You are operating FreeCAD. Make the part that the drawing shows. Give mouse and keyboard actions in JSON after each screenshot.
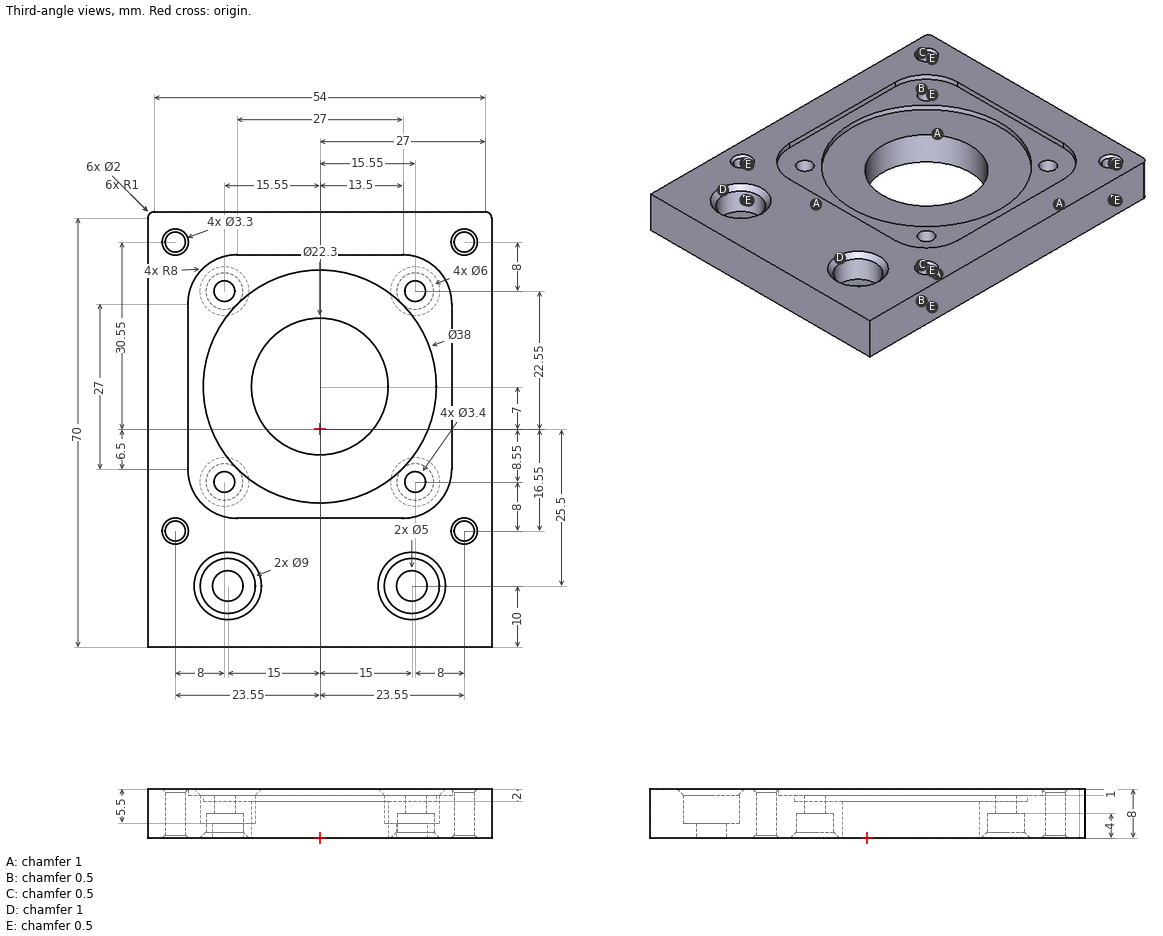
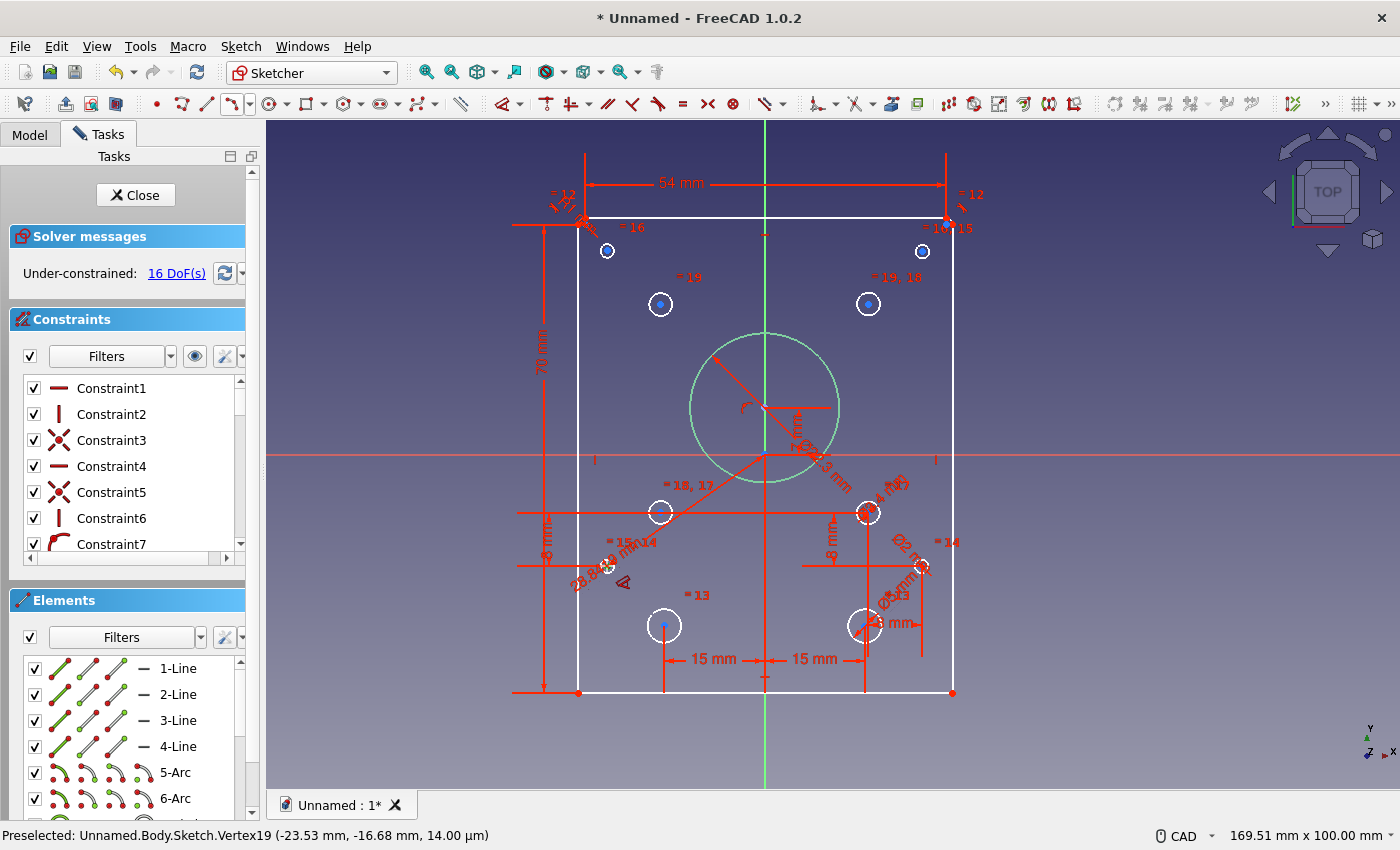
{"action": "left_click", "coordinate": [661, 512]}
{"action": "left_click", "coordinate": [634, 600]}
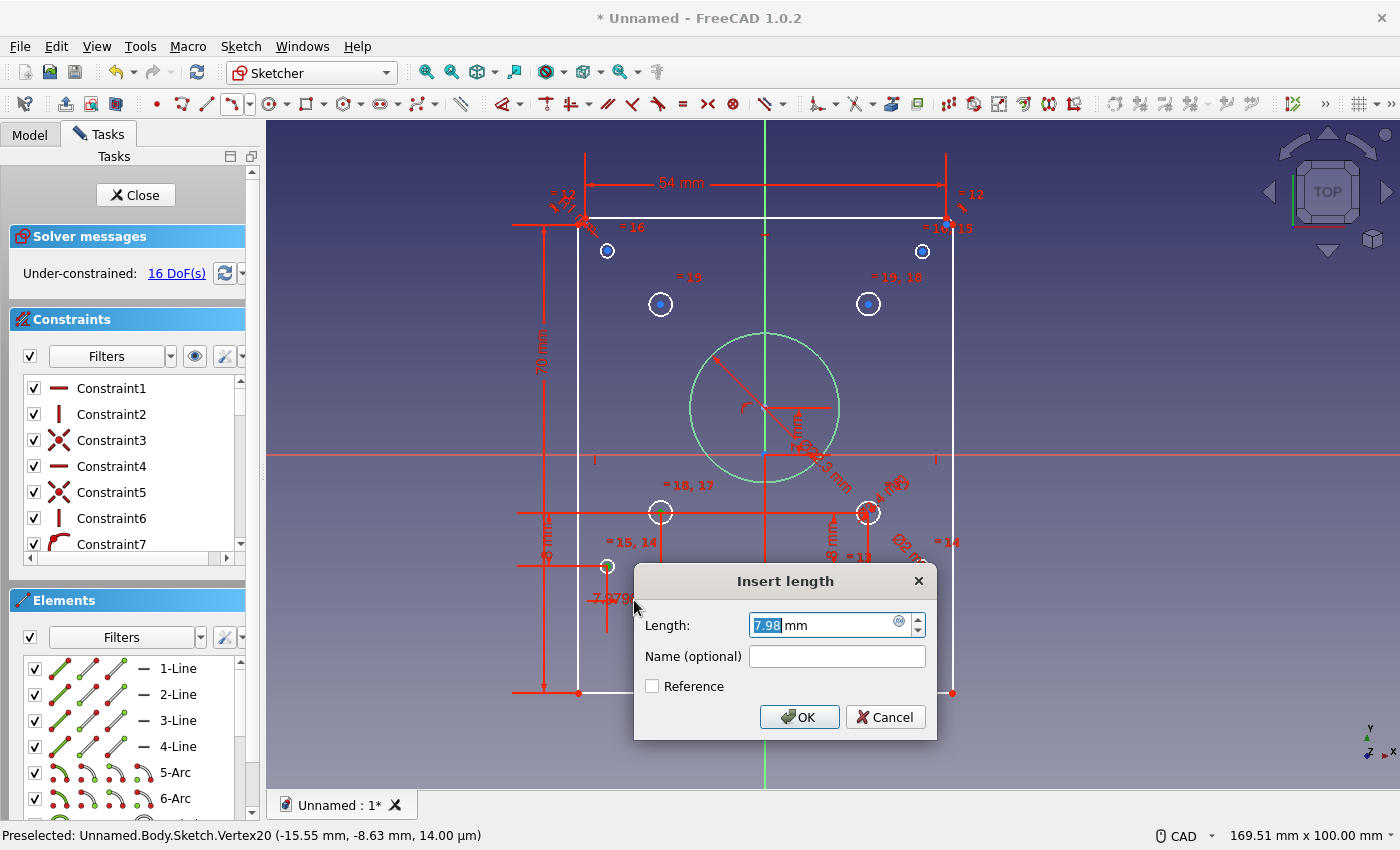
{"action": "type", "text": "8"}
{"action": "key", "text": "Return"}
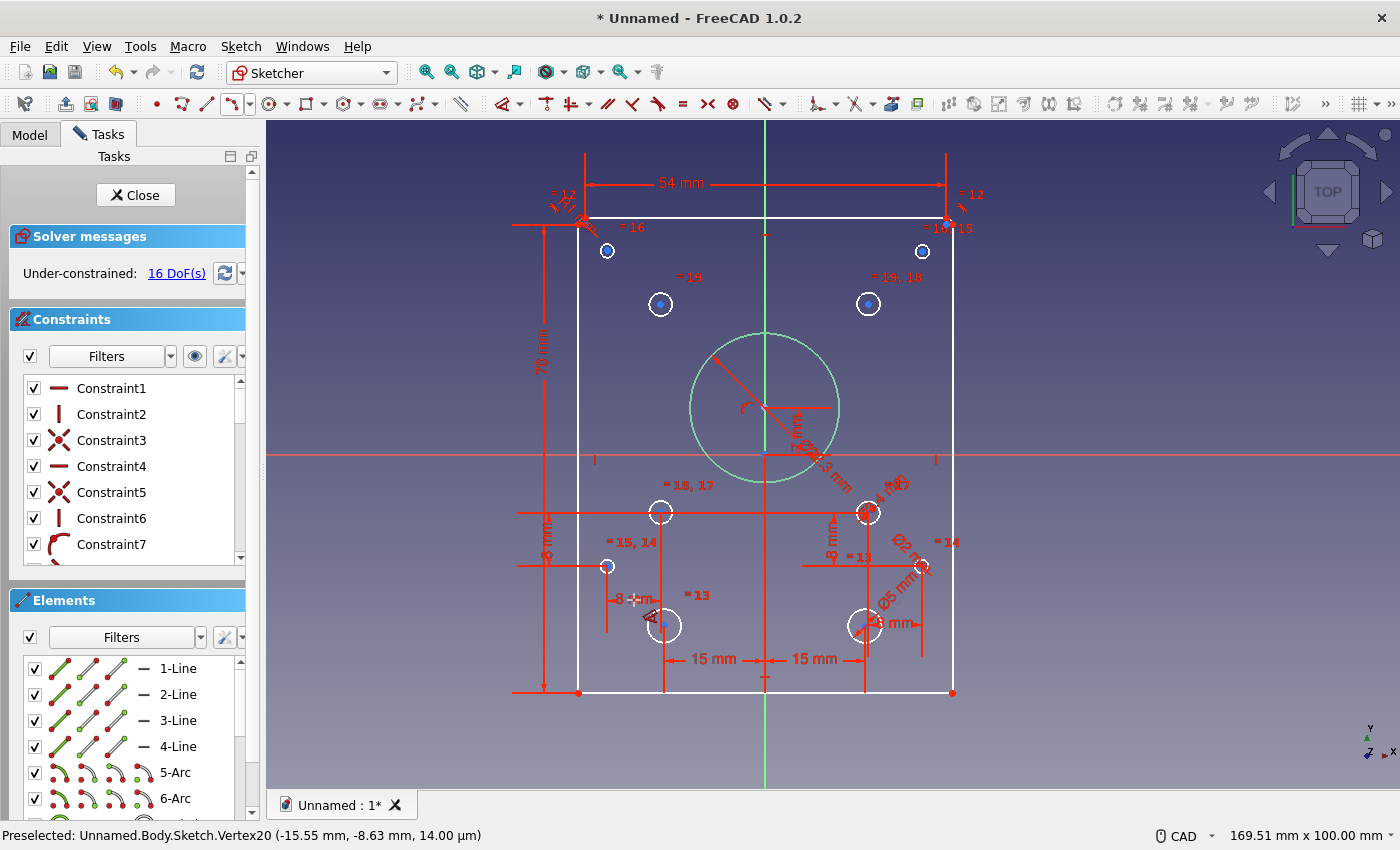
{"action": "left_click", "coordinate": [607, 566]}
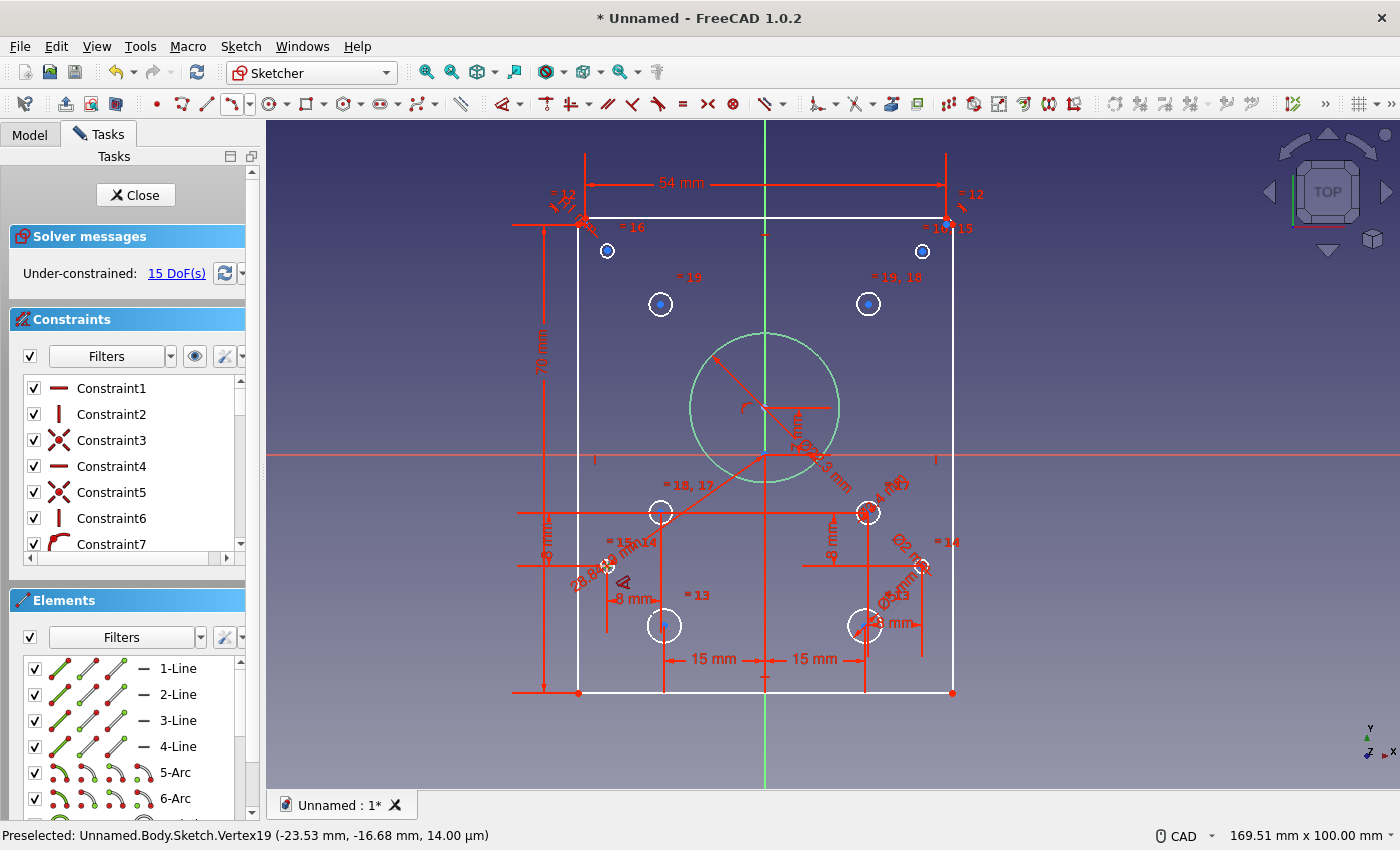
{"action": "left_click", "coordinate": [661, 512]}
{"action": "left_click", "coordinate": [695, 539]}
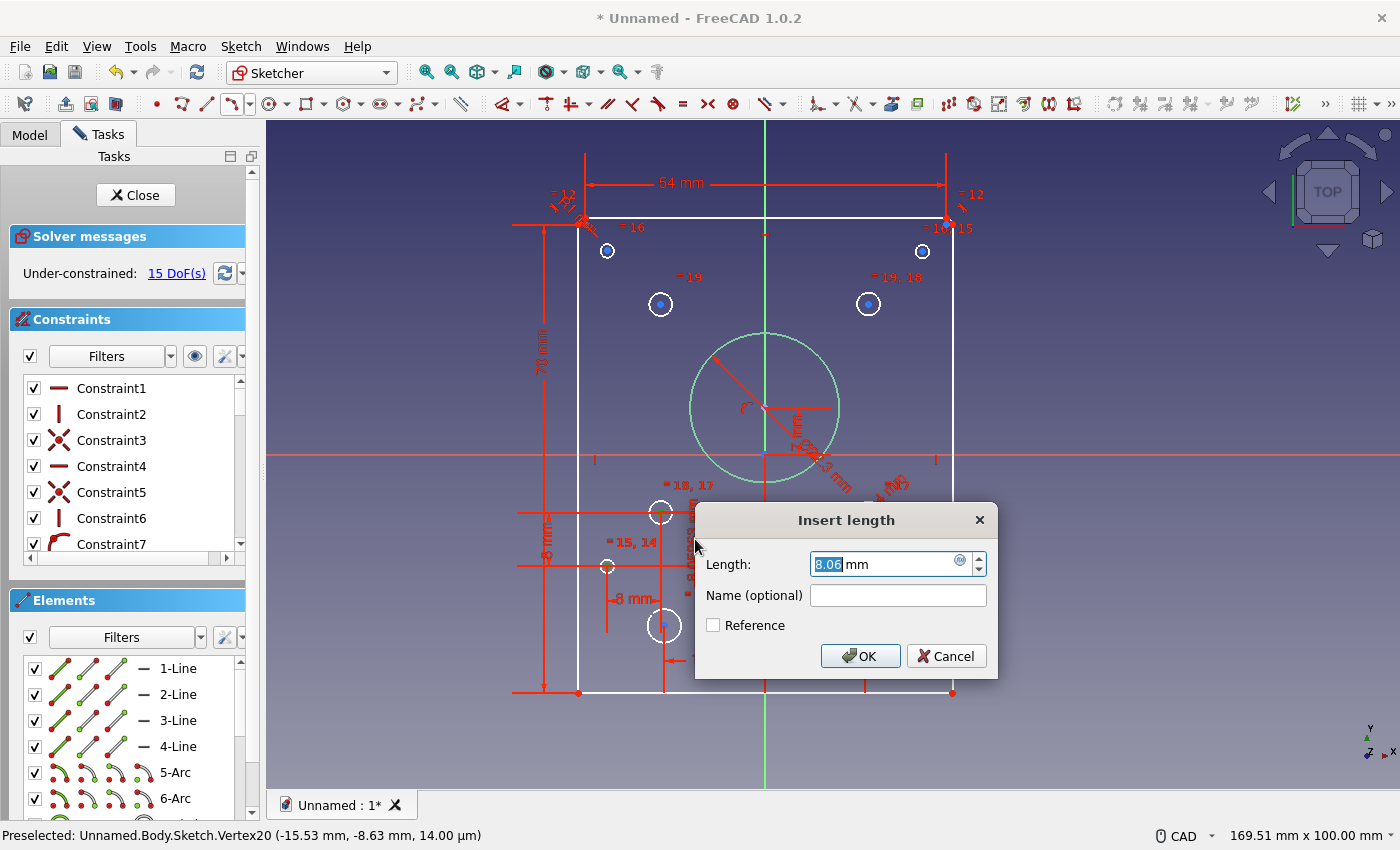
{"action": "type", "text": "8"}
{"action": "key", "text": "Return"}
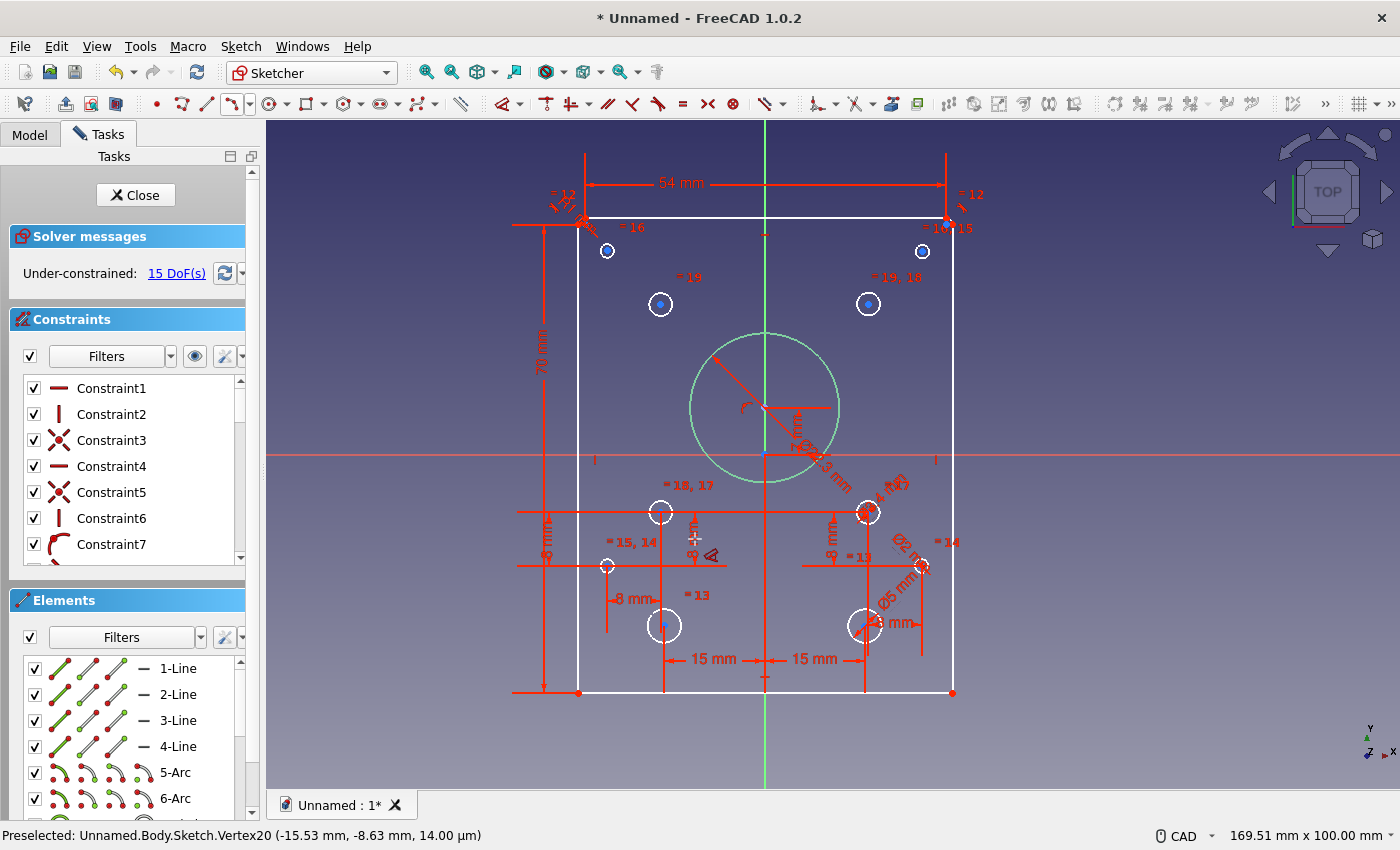
{"action": "left_click", "coordinate": [922, 566]}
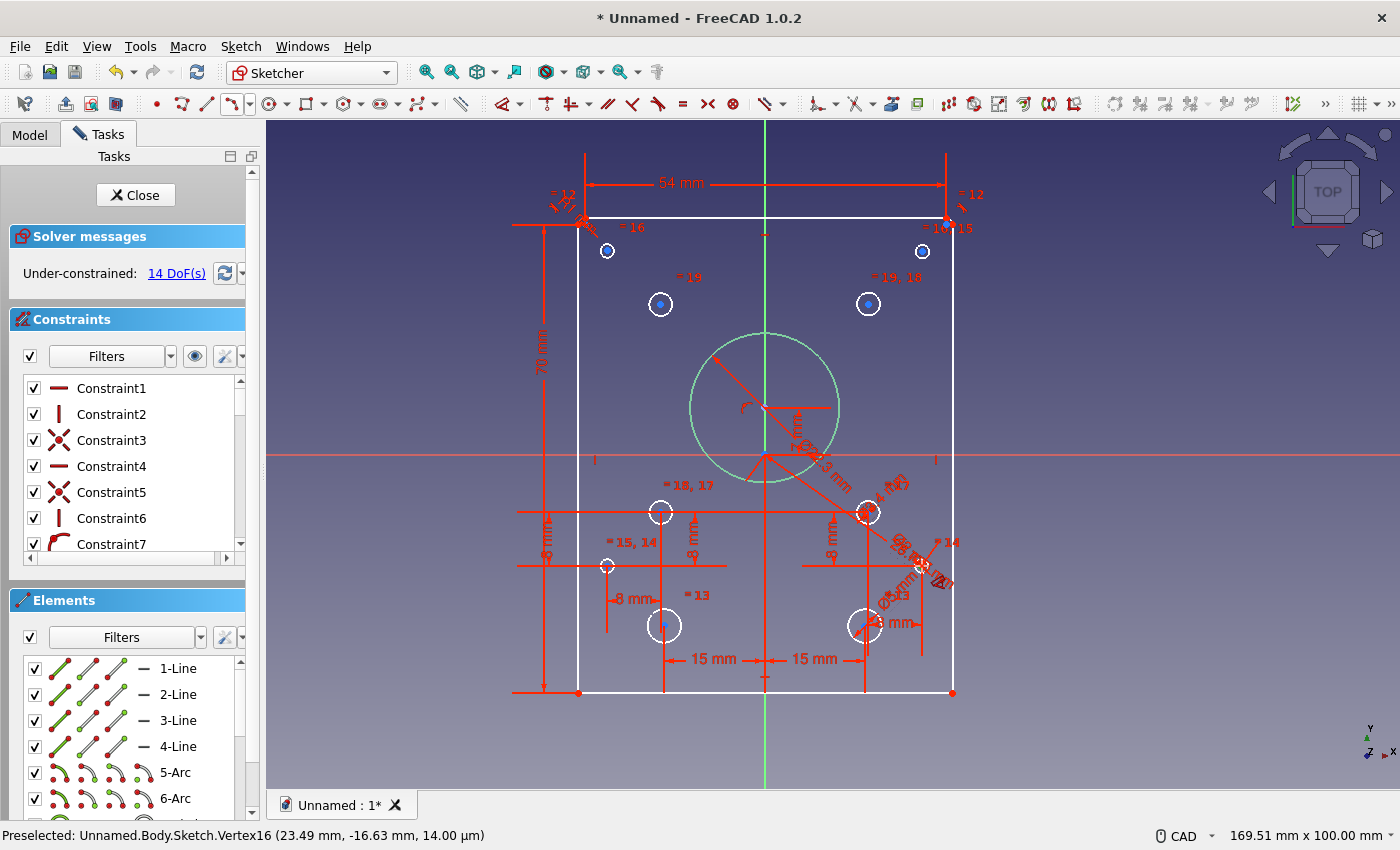
{"action": "left_click", "coordinate": [869, 304]}
{"action": "left_click", "coordinate": [895, 270]}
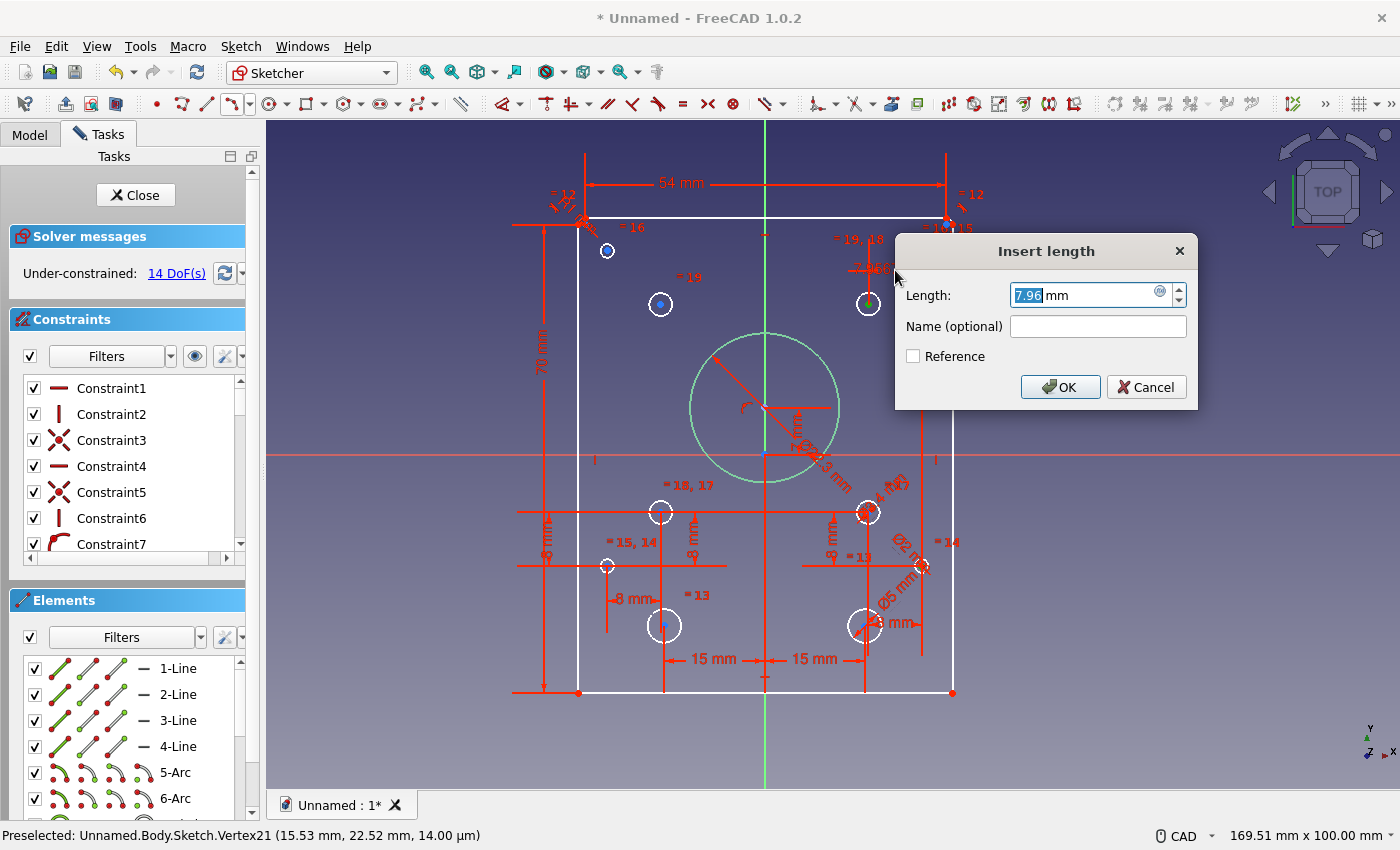
{"action": "type", "text": "8"}
{"action": "key", "text": "Return"}